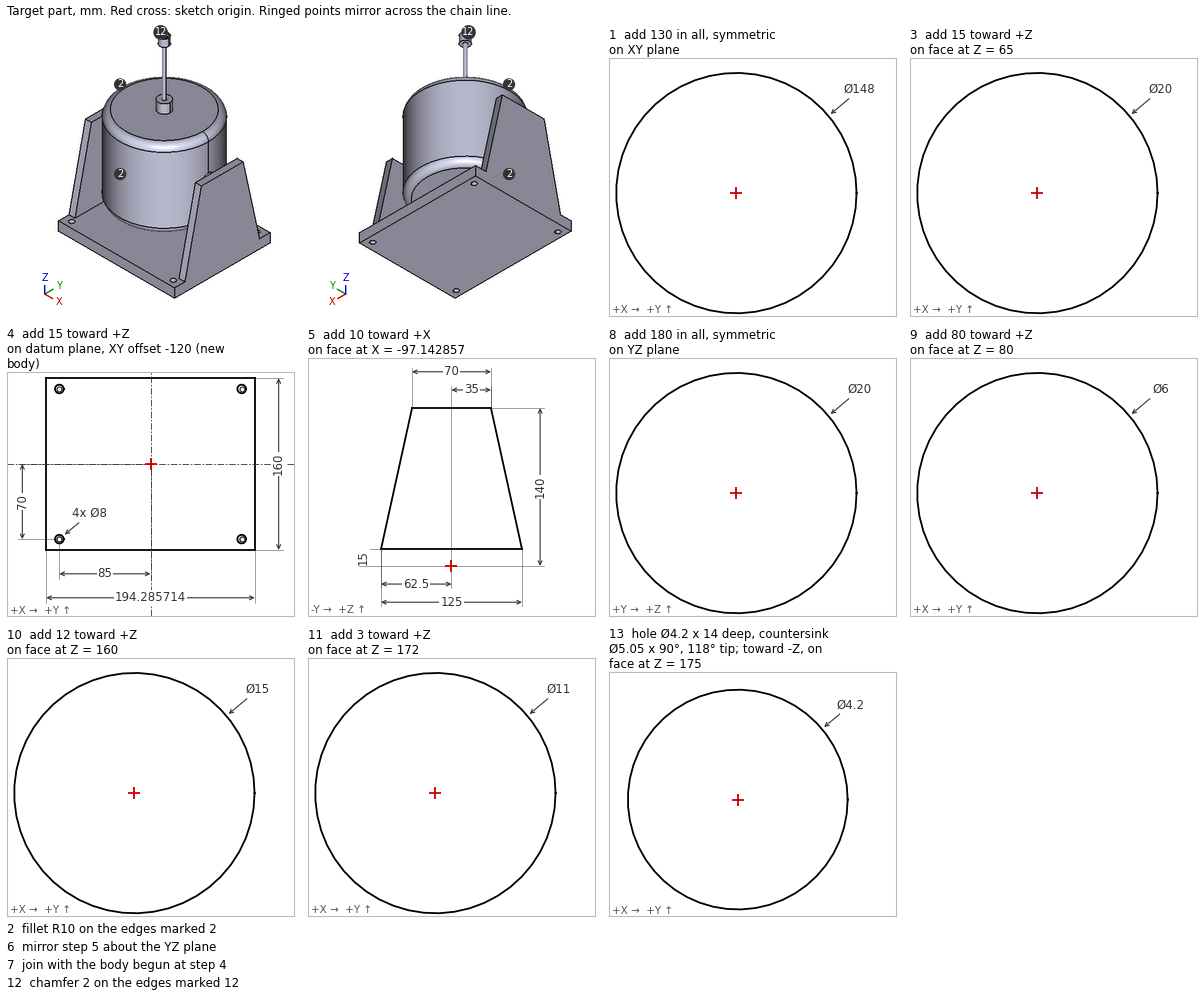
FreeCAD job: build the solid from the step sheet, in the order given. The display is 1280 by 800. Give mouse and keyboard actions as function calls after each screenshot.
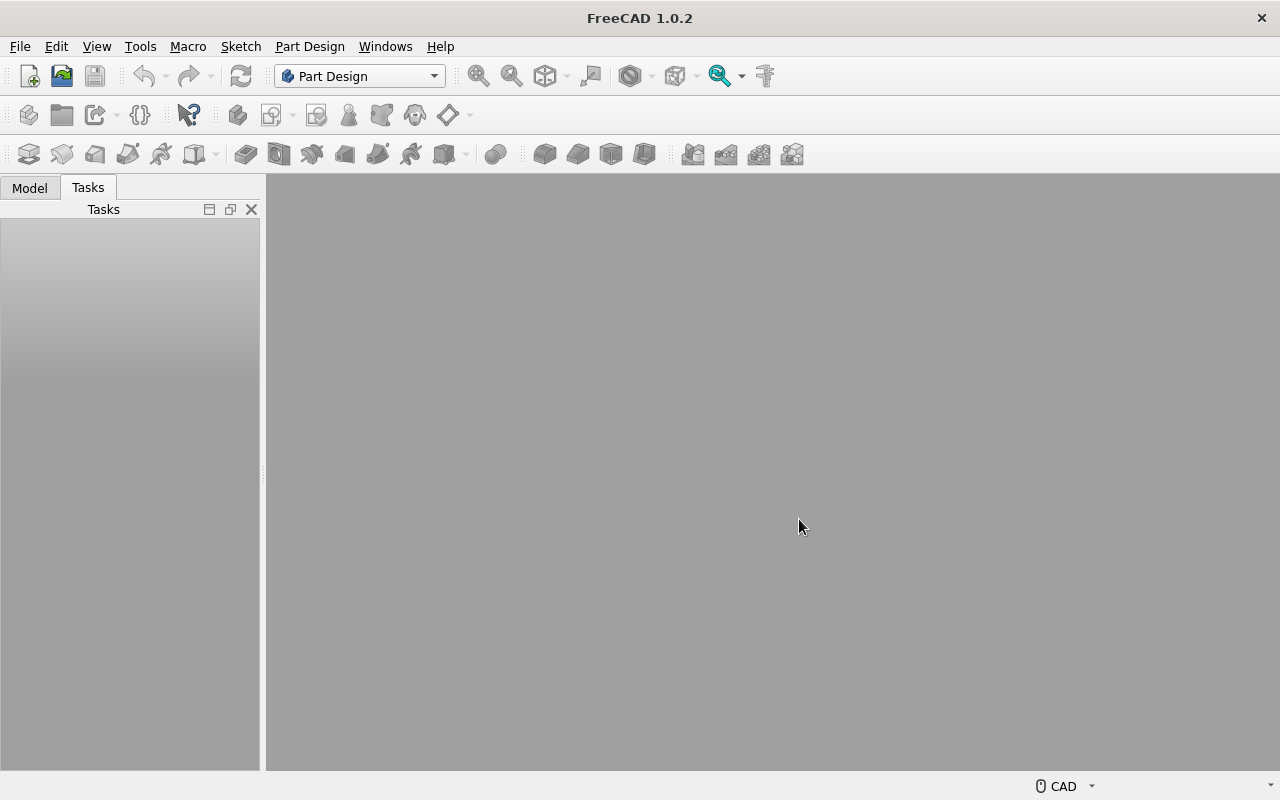
key(ctrl+n)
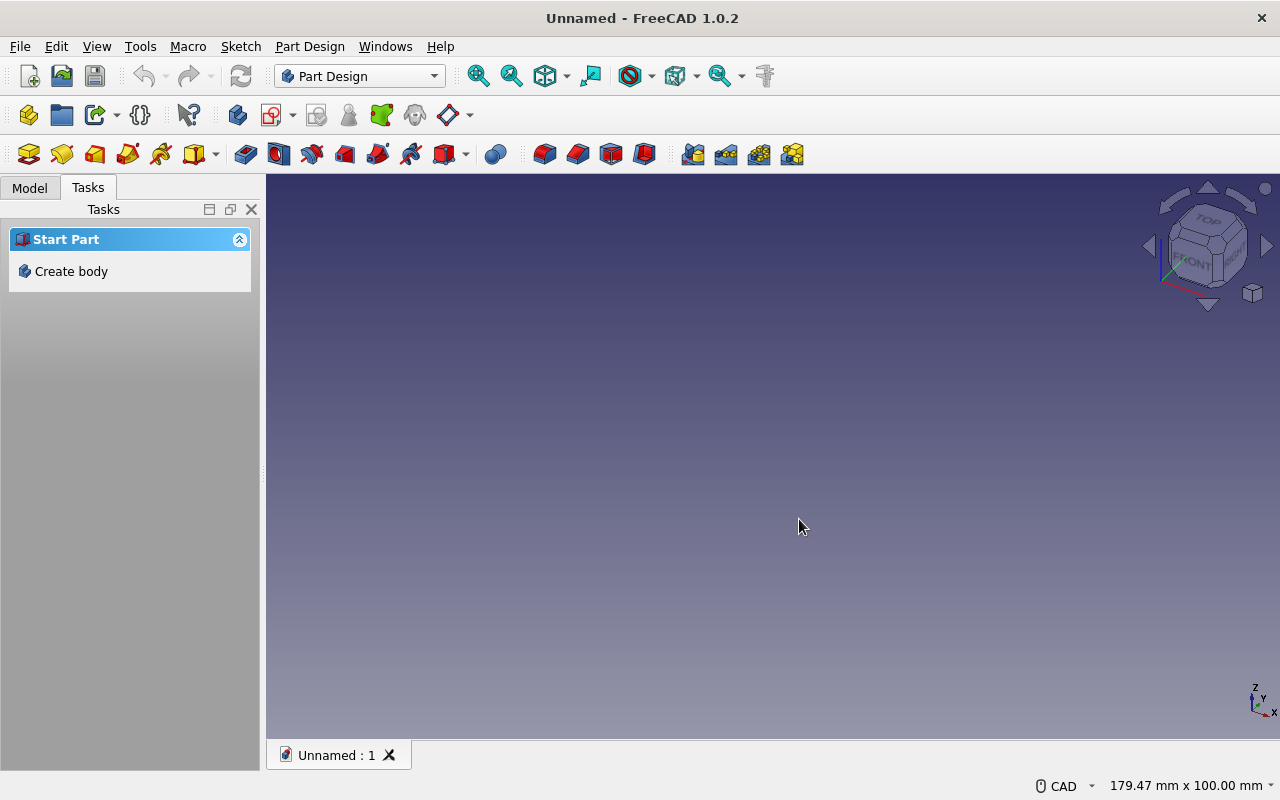
click(270, 116)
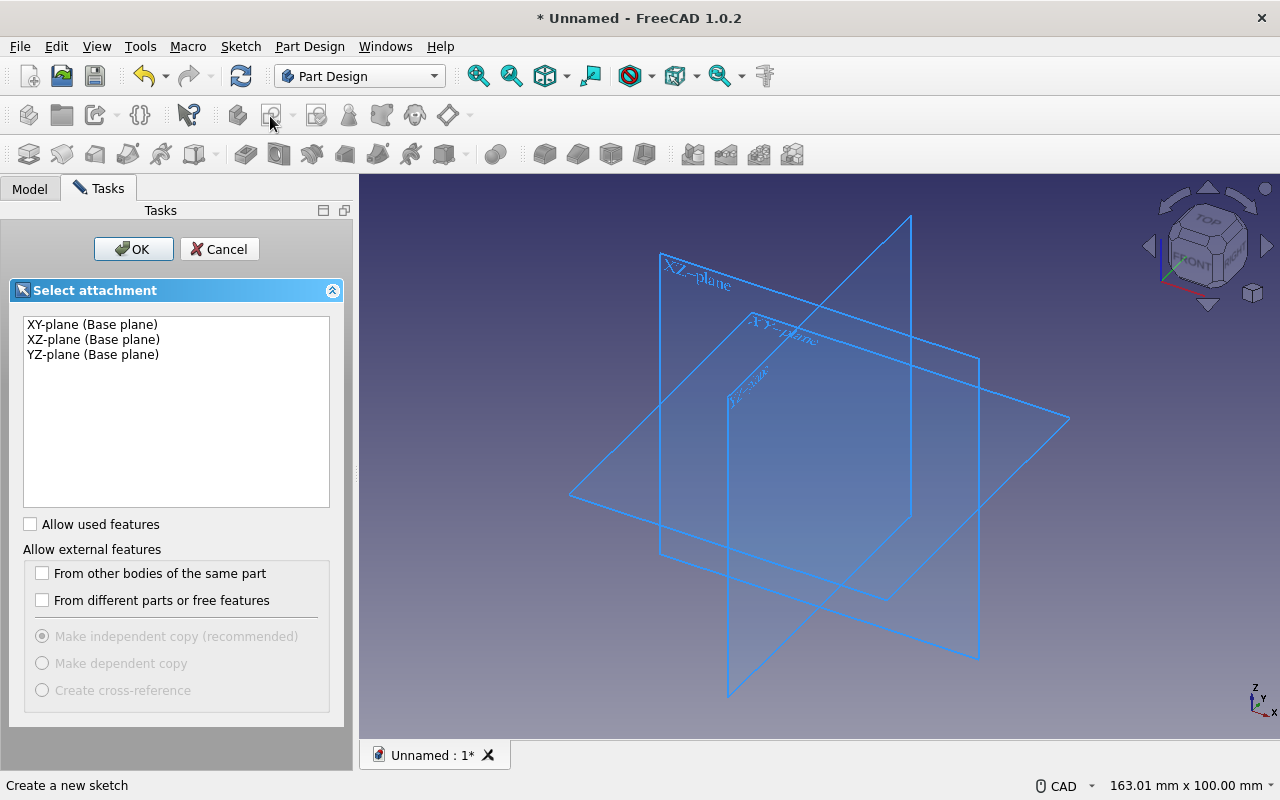
click(84, 324)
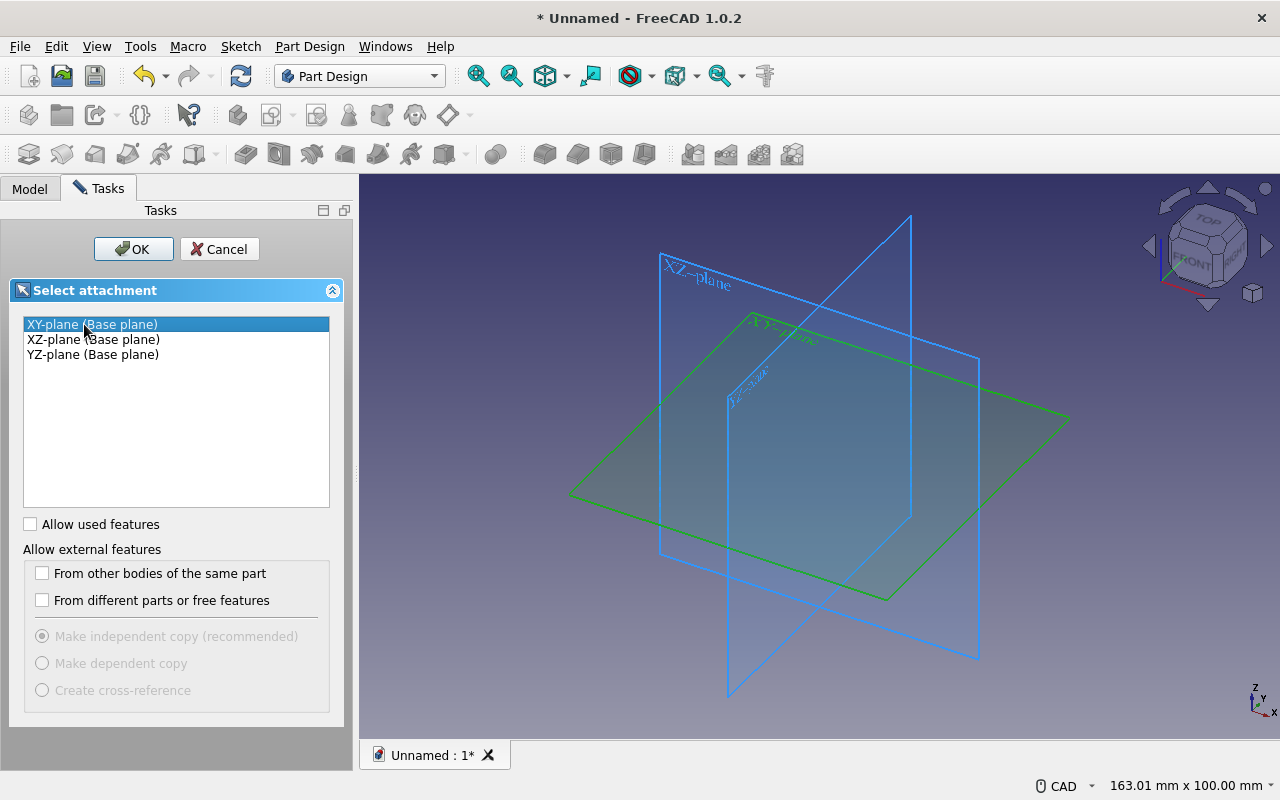
click(134, 249)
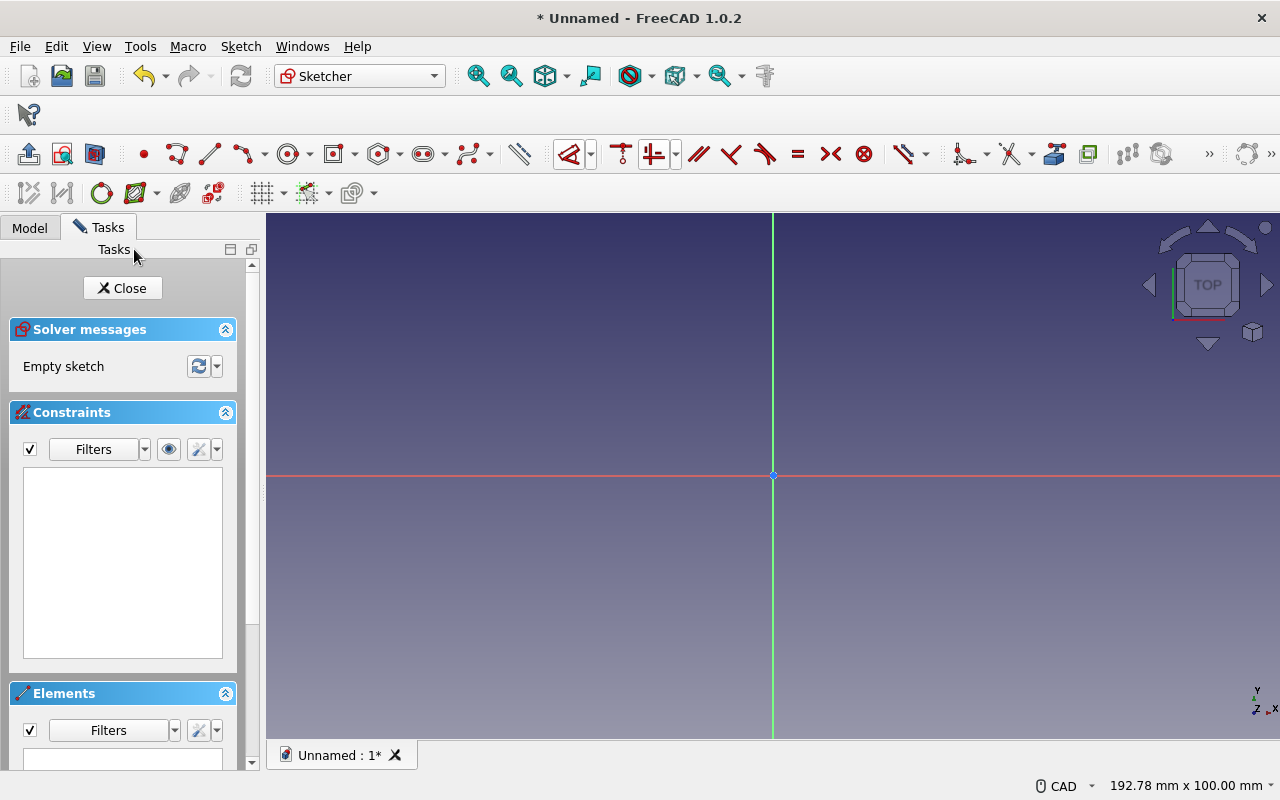
scroll(649, 476, down, 4)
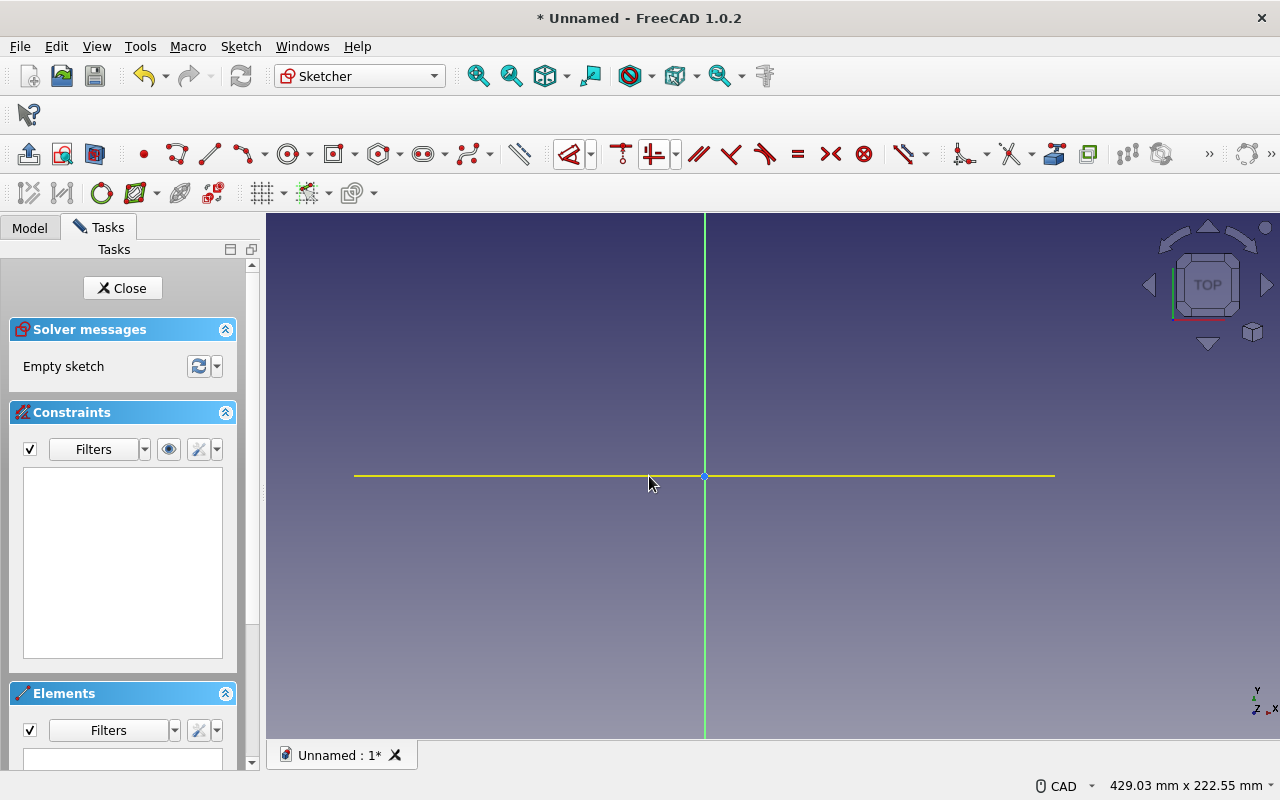
key(g)
key(c)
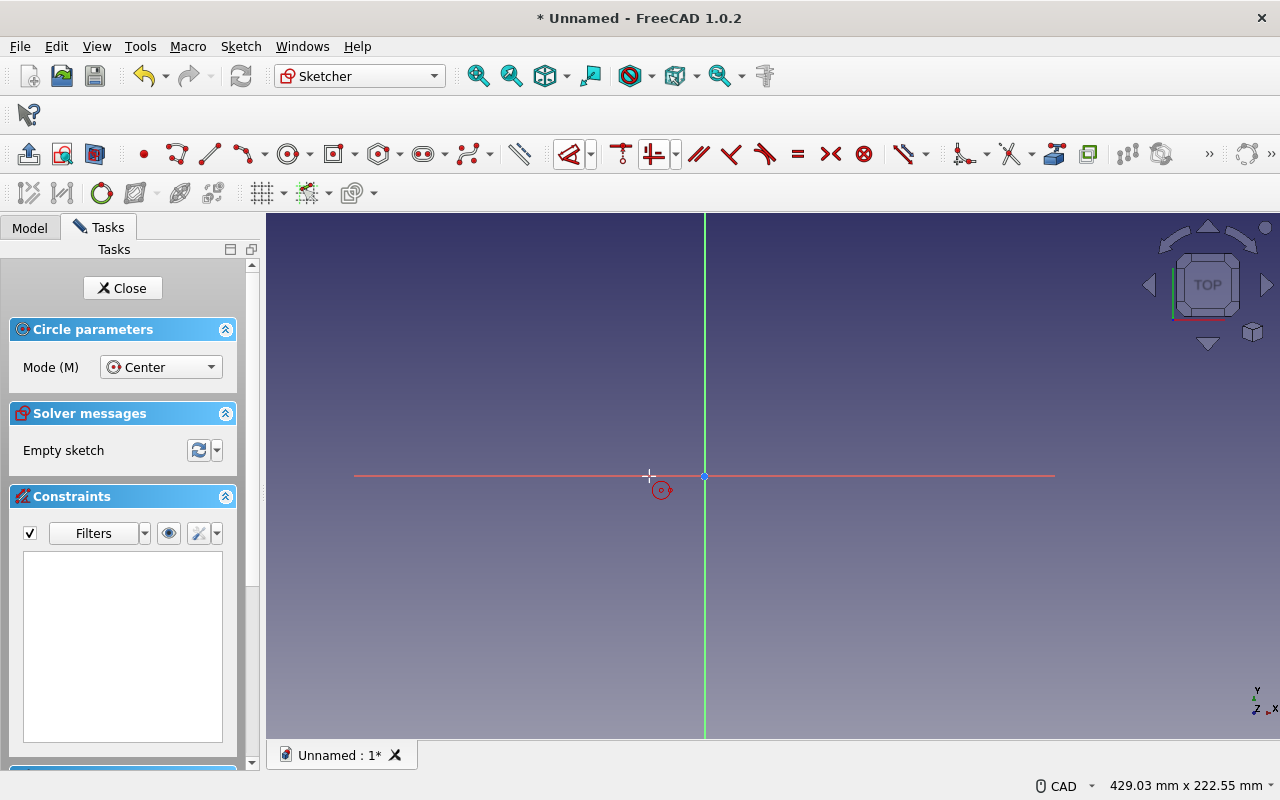
click(705, 476)
click(829, 353)
key(Escape)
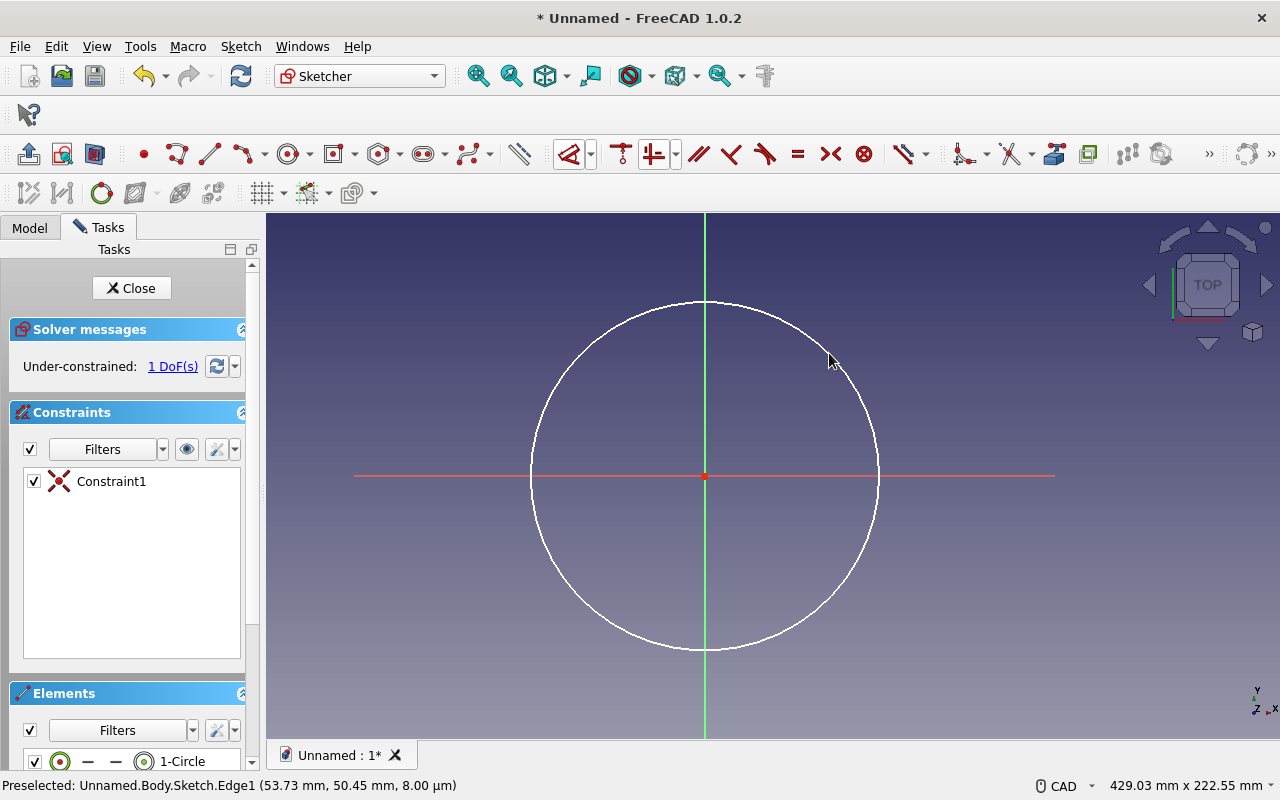
click(828, 353)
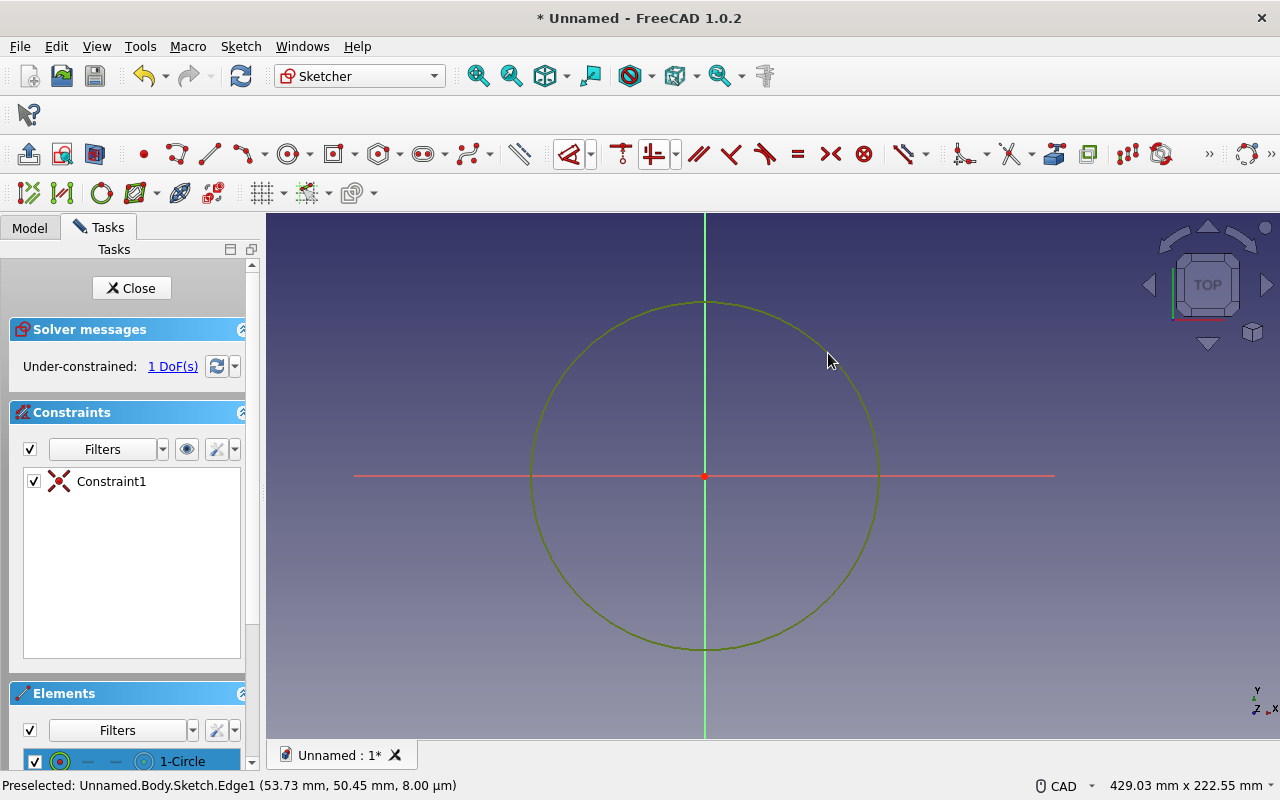
click(590, 154)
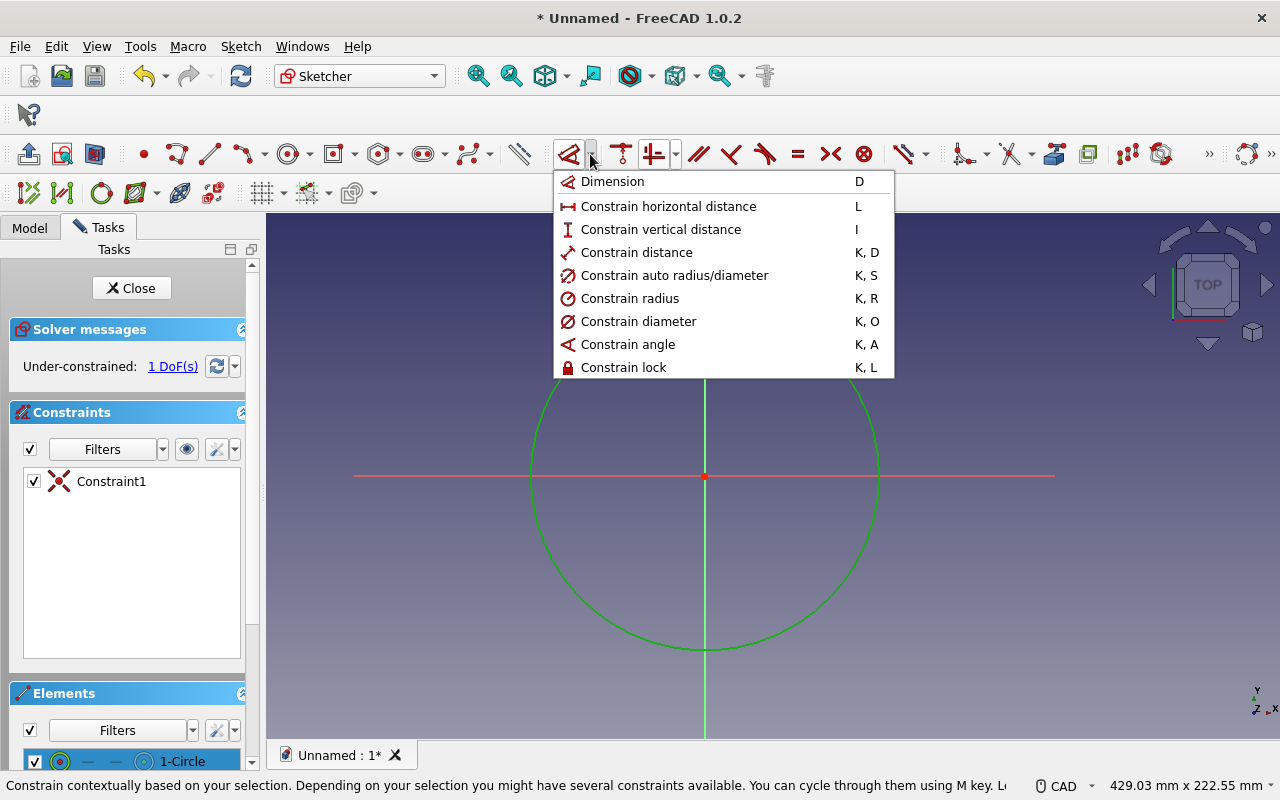
click(724, 322)